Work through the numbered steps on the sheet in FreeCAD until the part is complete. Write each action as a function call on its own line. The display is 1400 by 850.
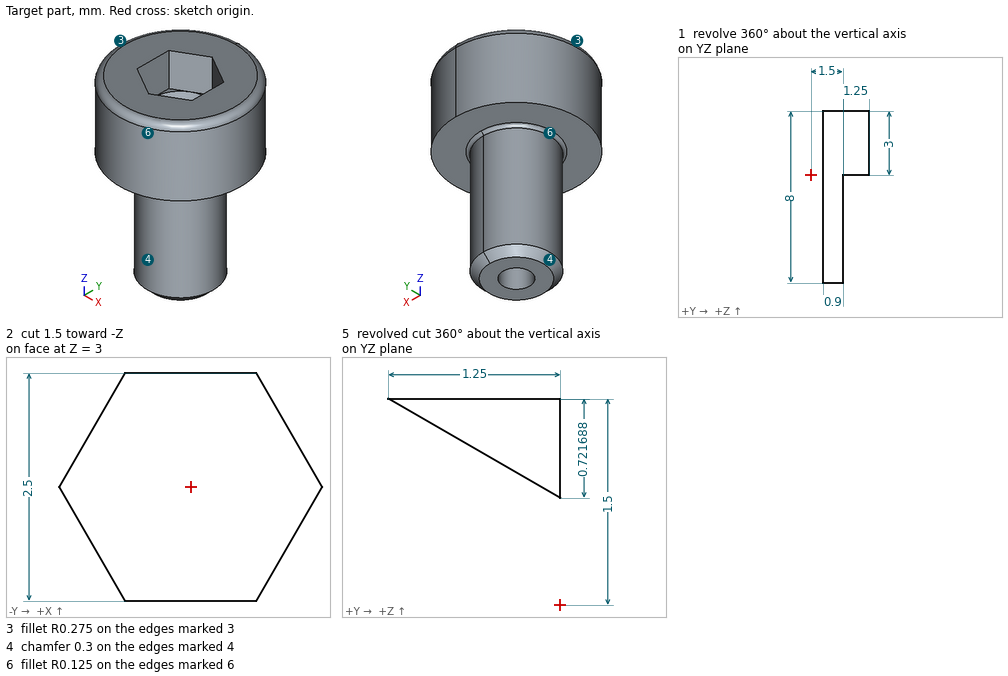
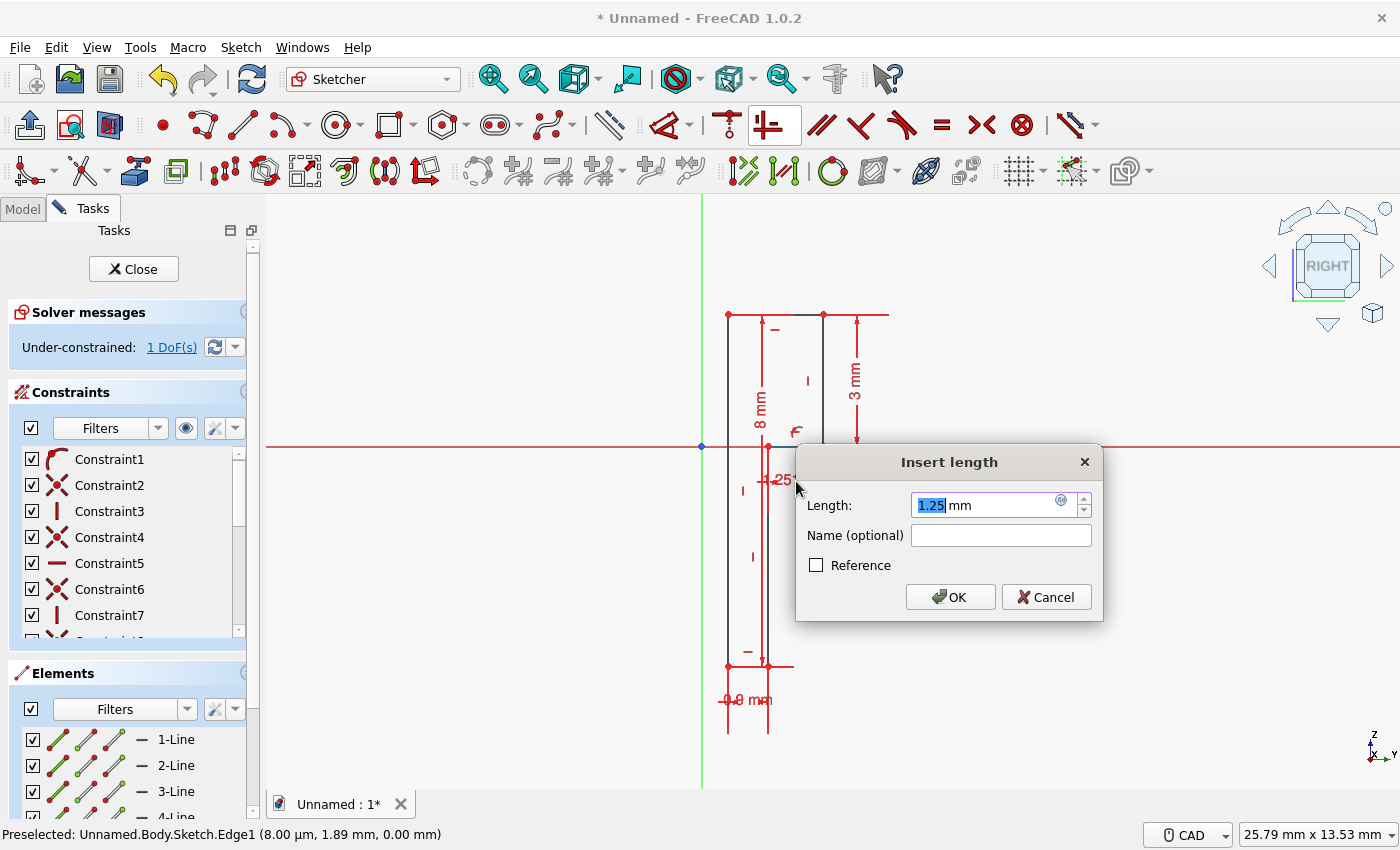
text(1.25)
key(Return)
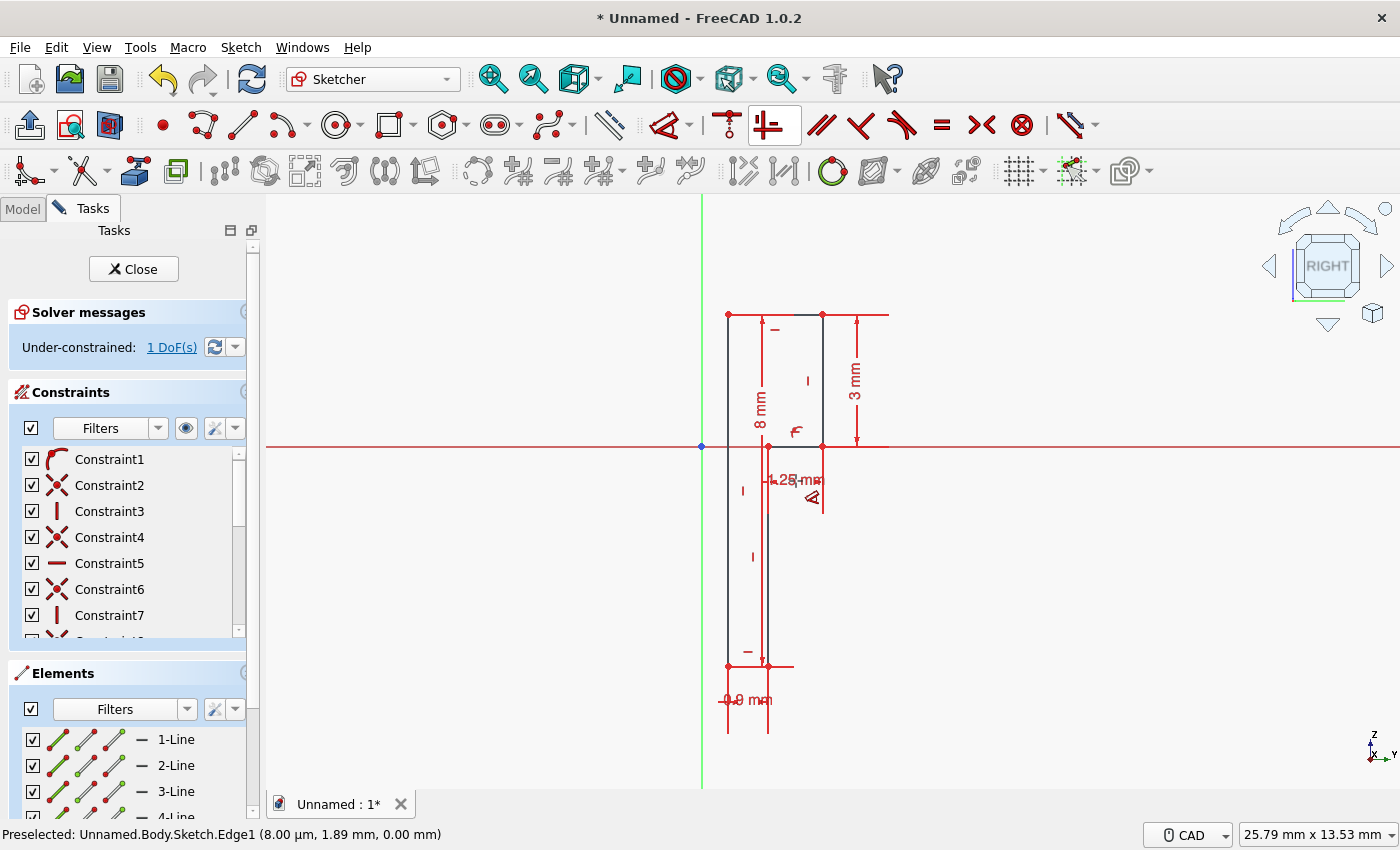
click(768, 447)
click(750, 389)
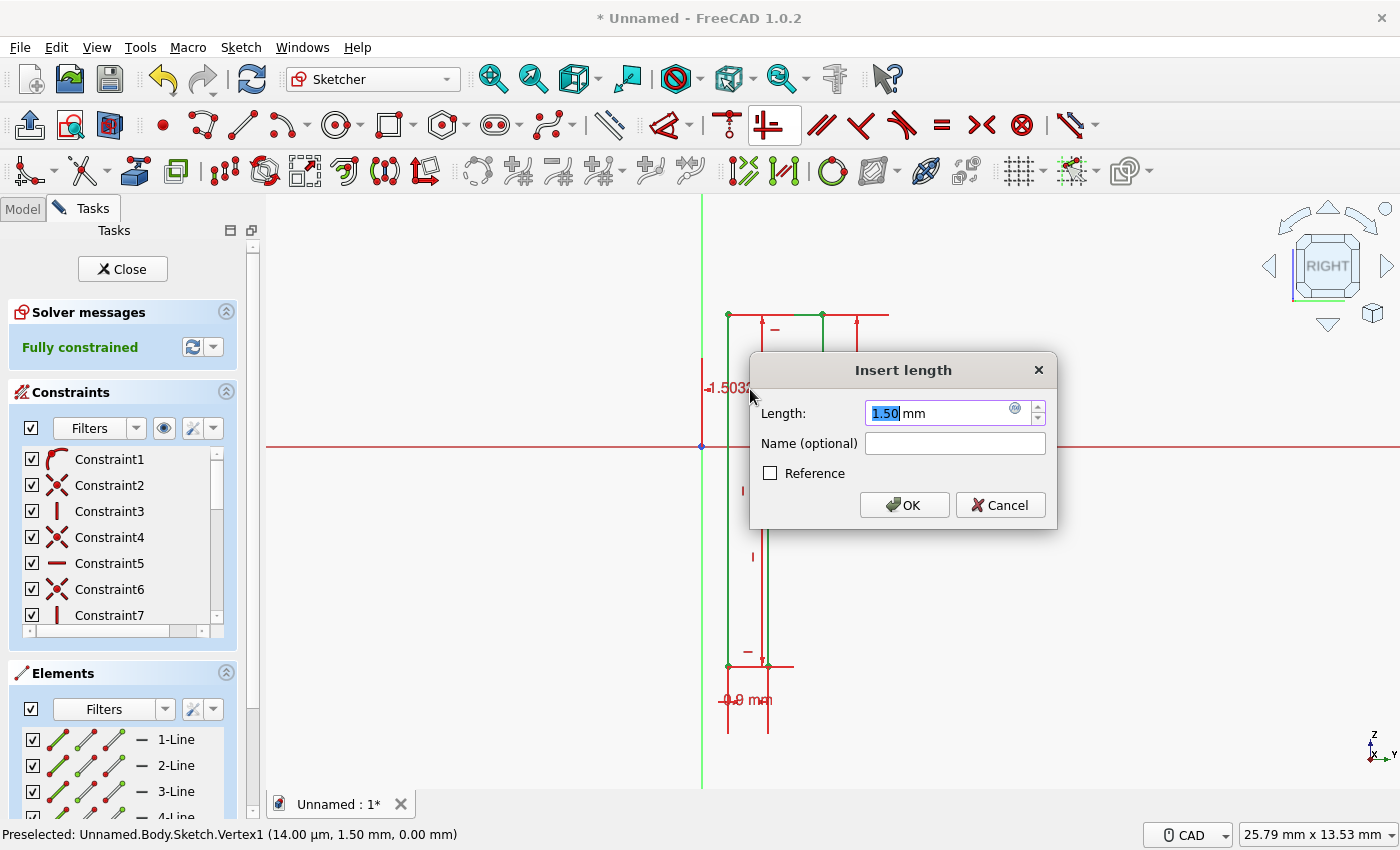
text(1.5)
key(Return)
key(Escape)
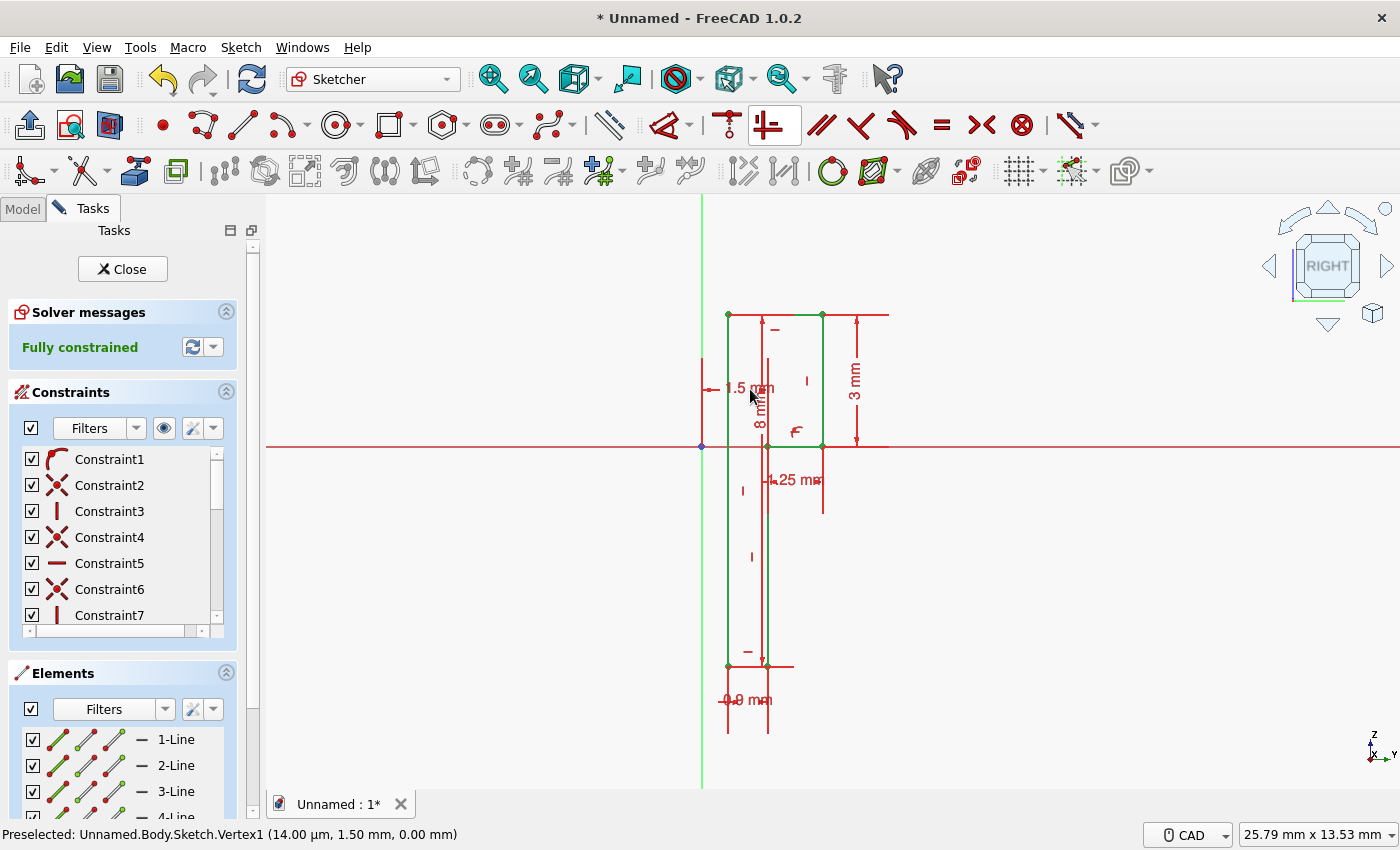
click(123, 269)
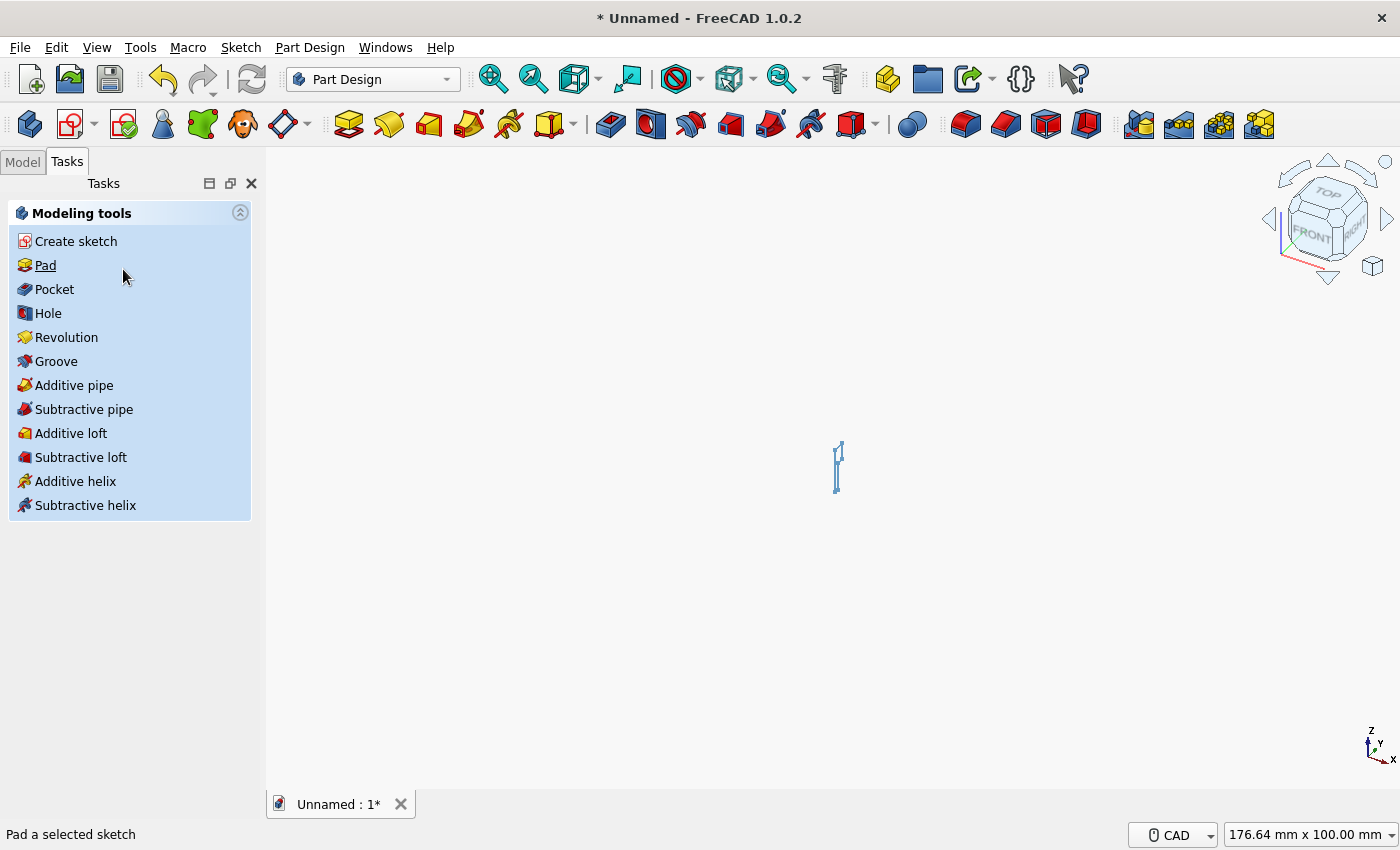
click(390, 124)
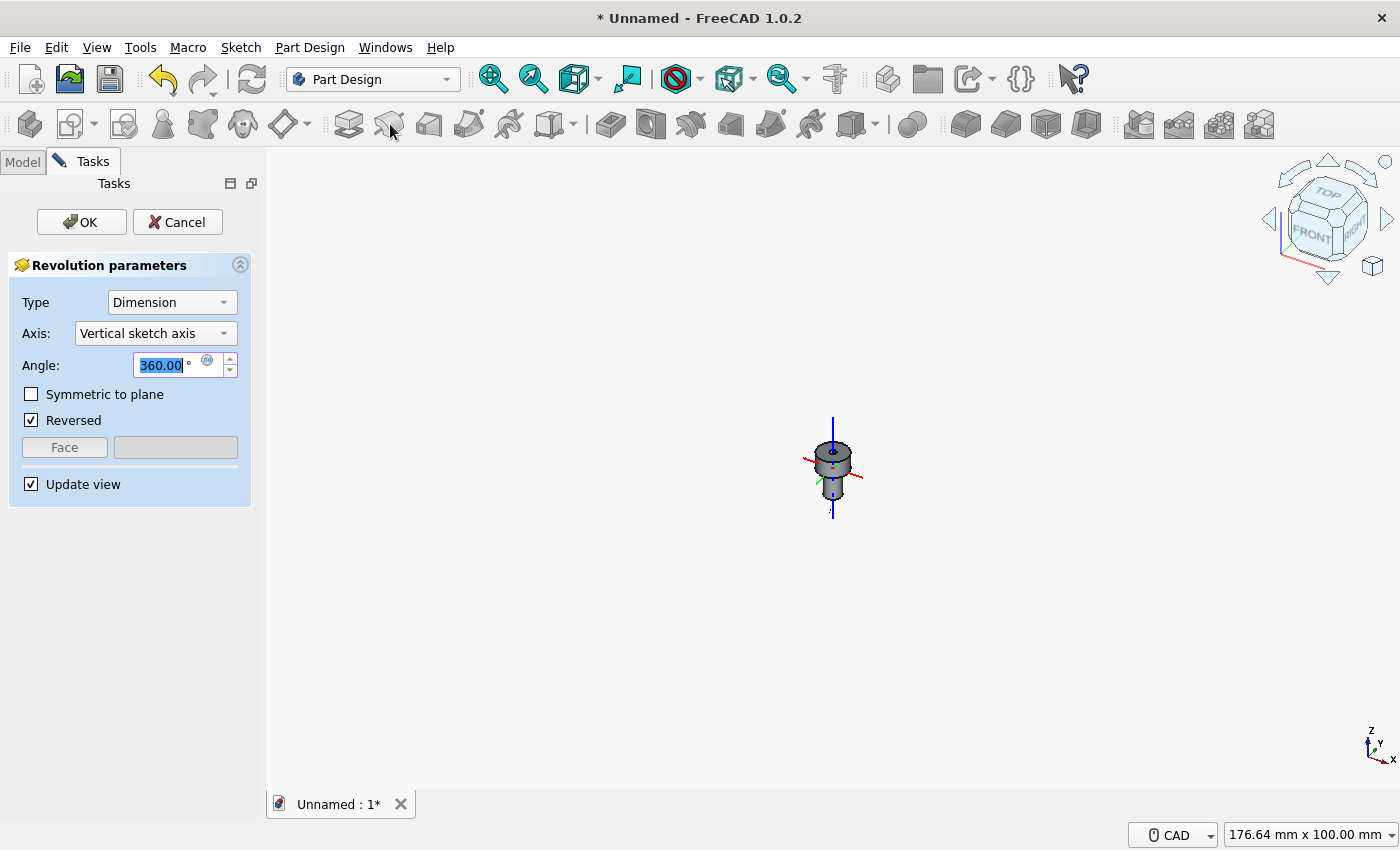
click(82, 222)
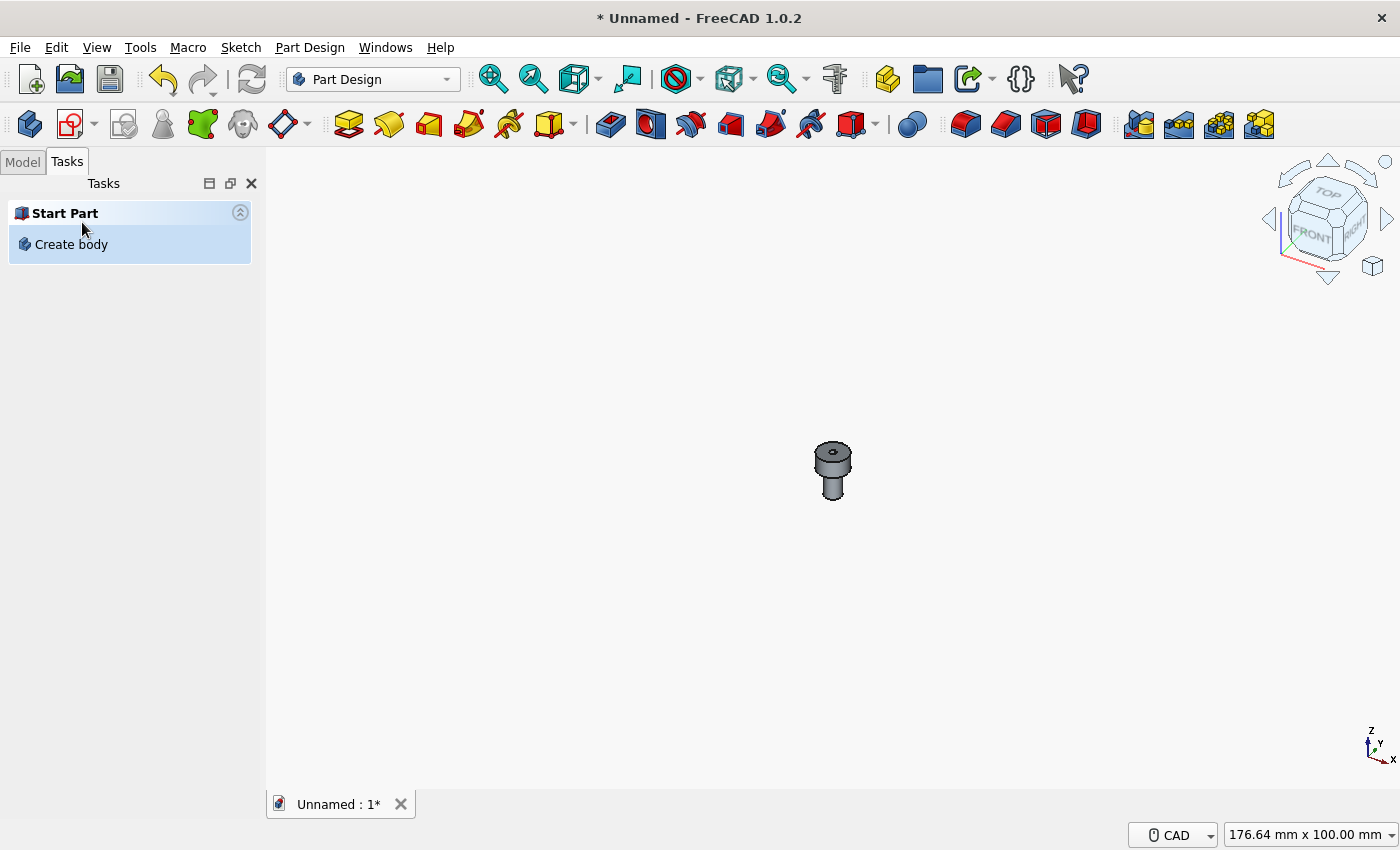
click(494, 80)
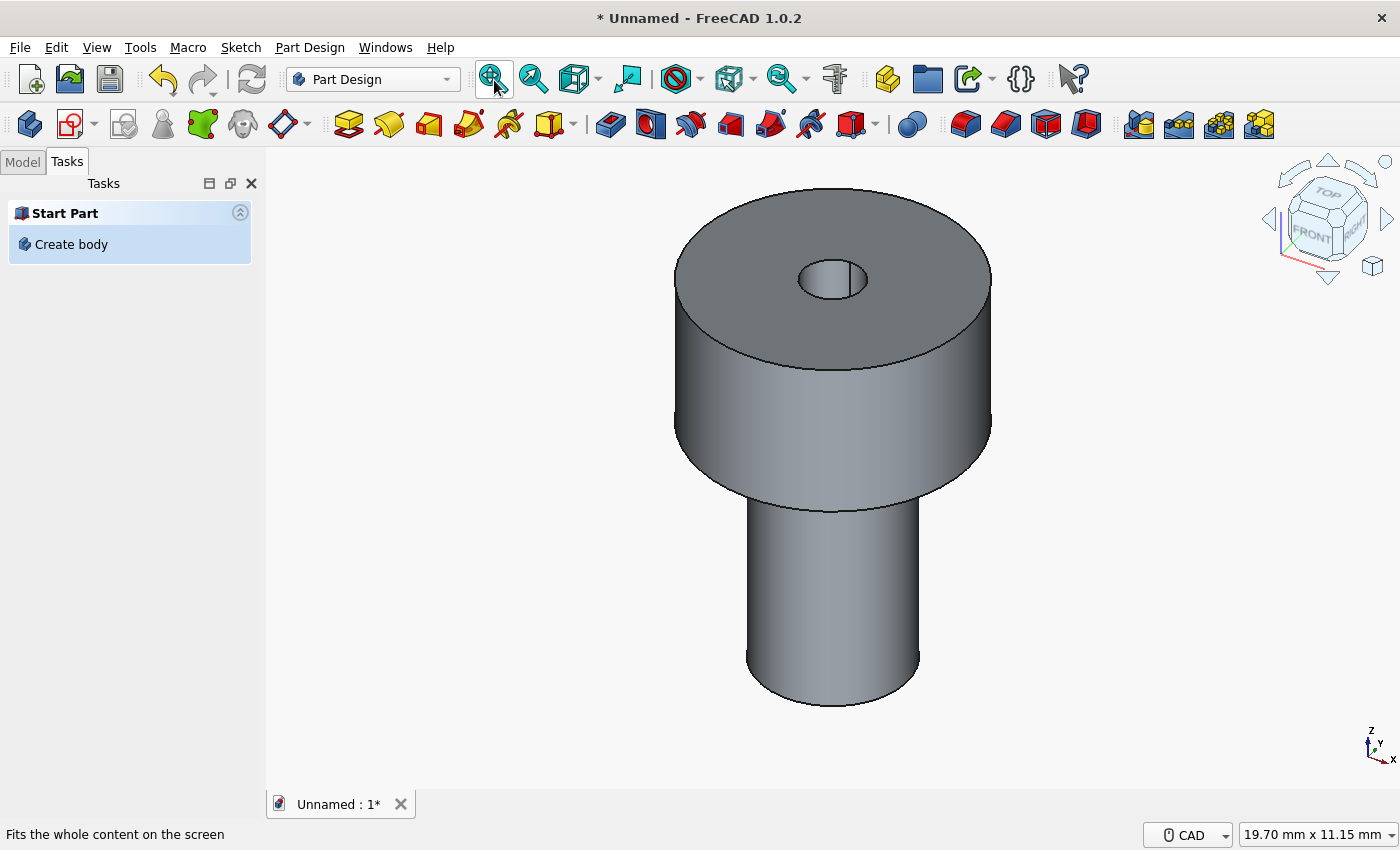
click(934, 282)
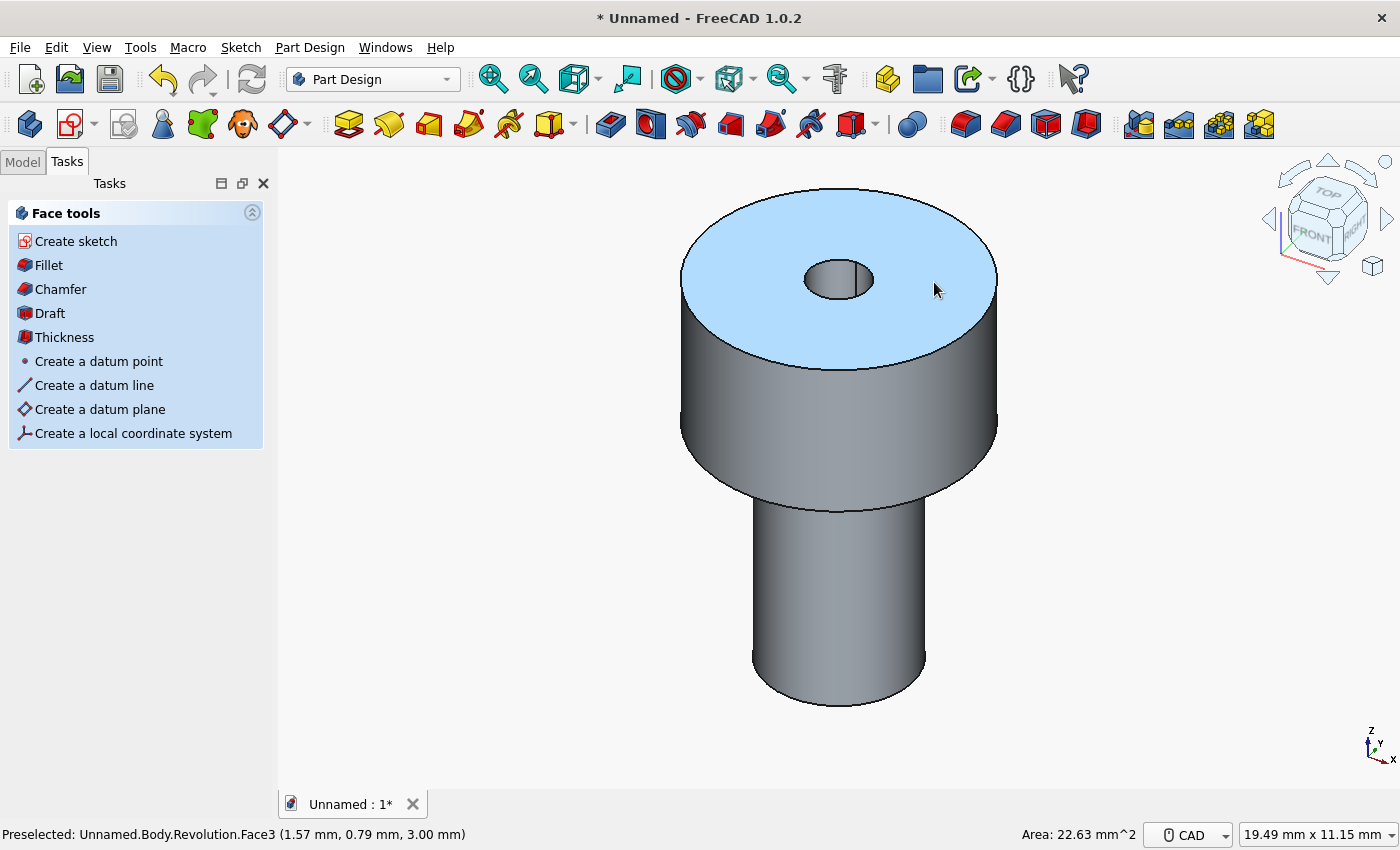
click(70, 124)